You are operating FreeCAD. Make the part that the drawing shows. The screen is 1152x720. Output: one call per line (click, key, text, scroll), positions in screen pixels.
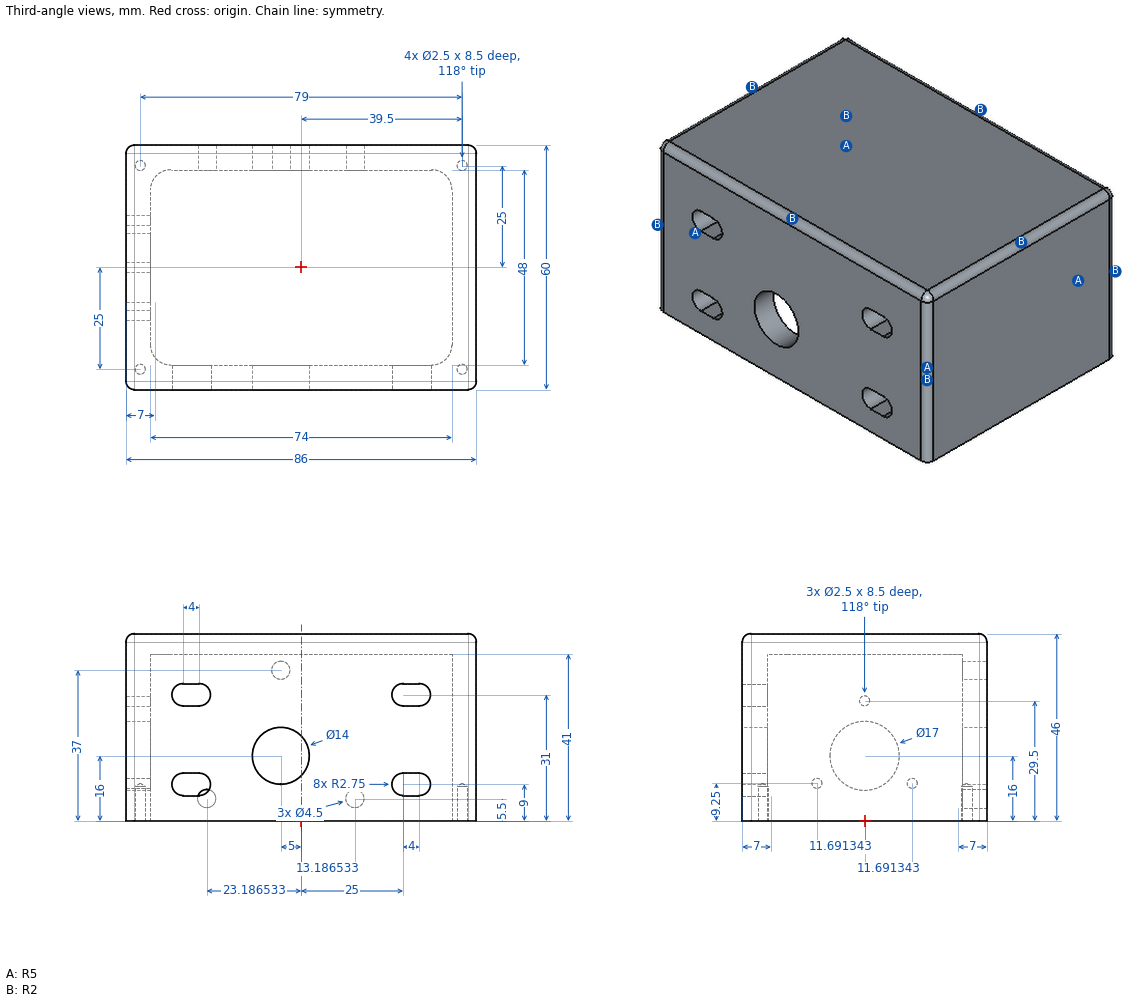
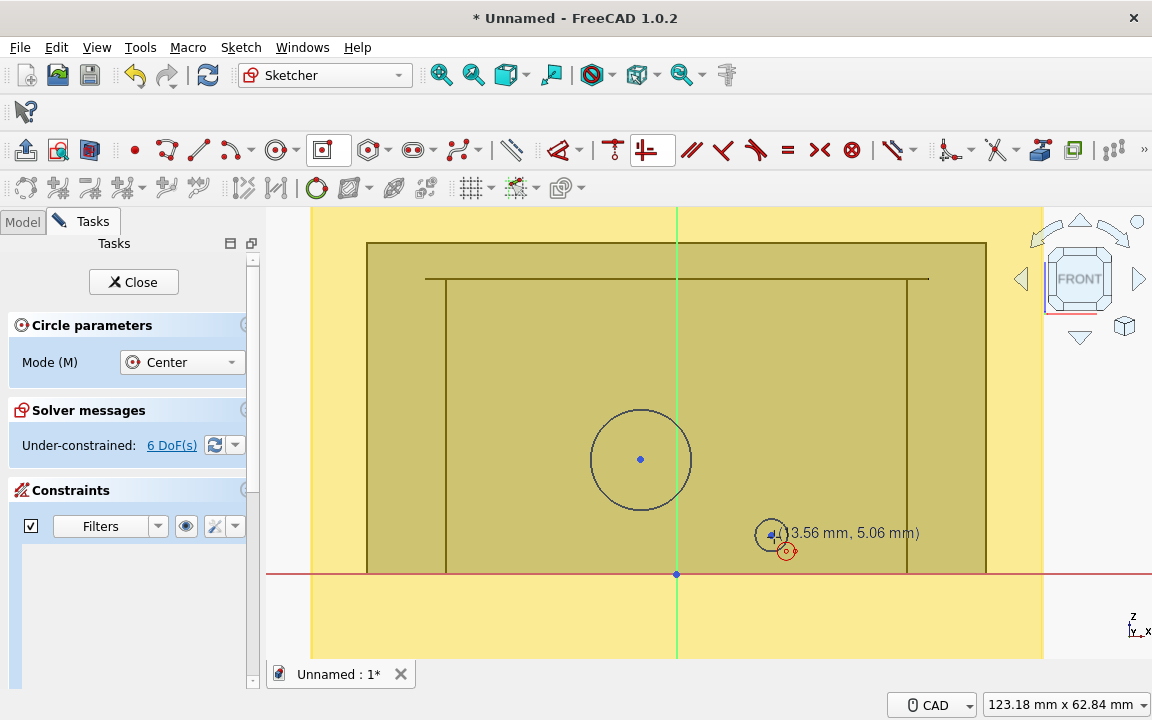
scroll(641, 308, up, 2)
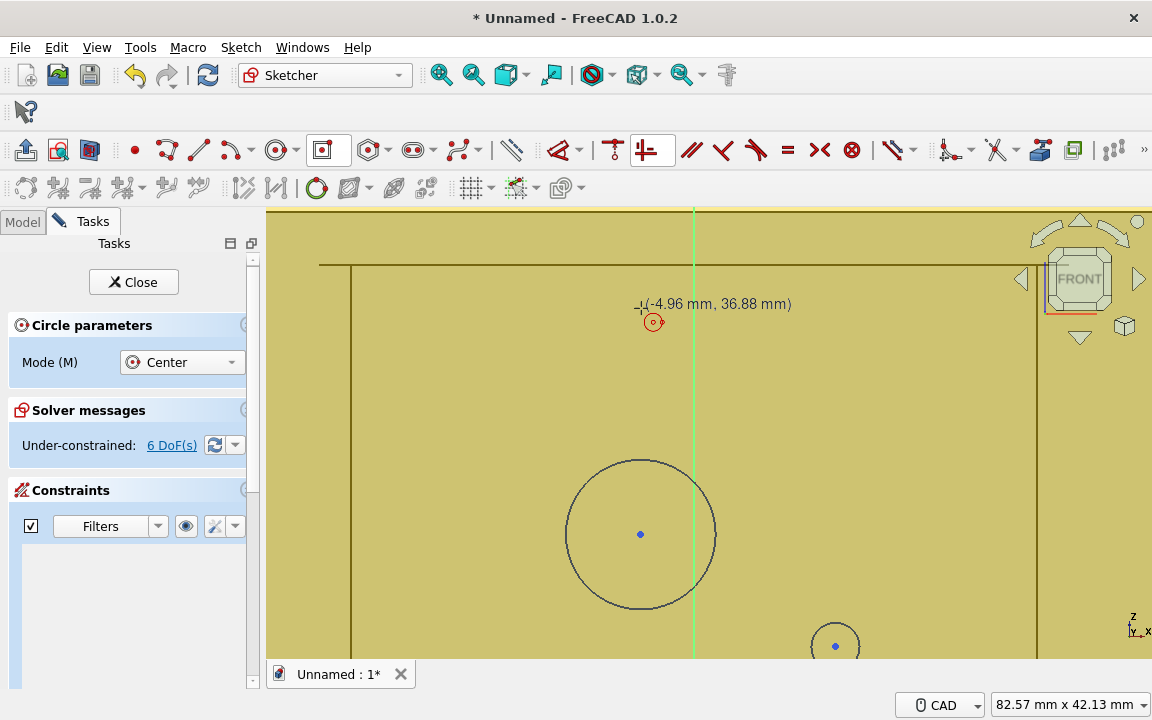
click(640, 308)
click(657, 291)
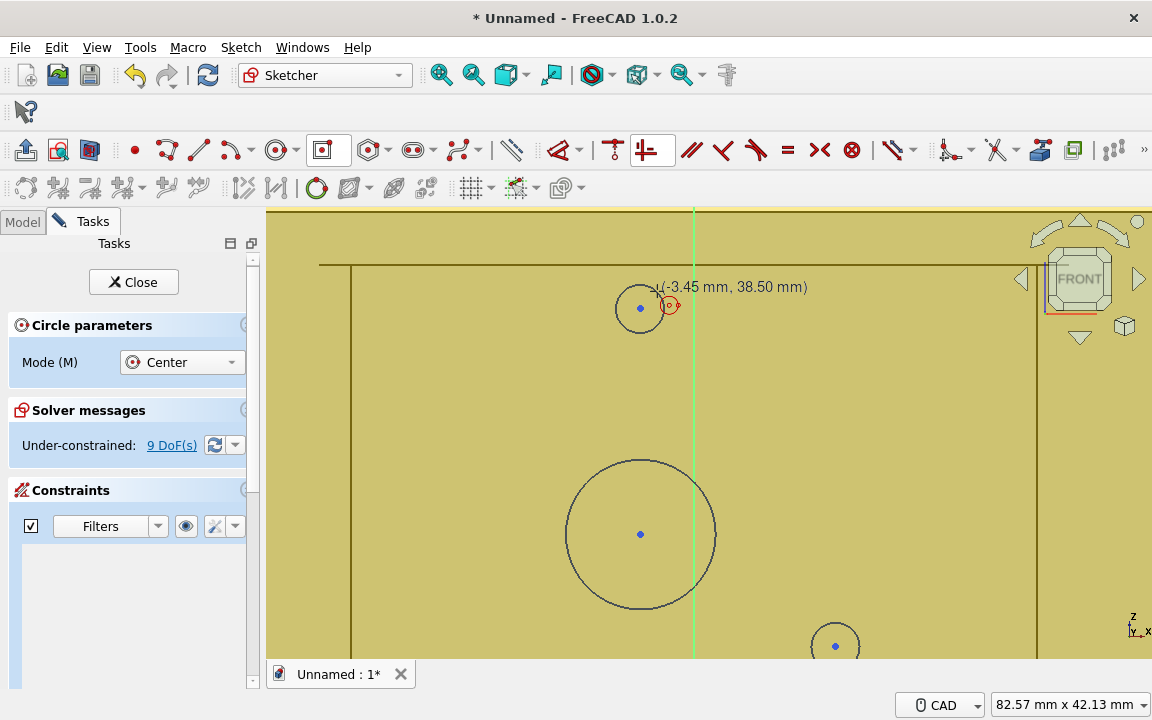
scroll(641, 308, down, 2)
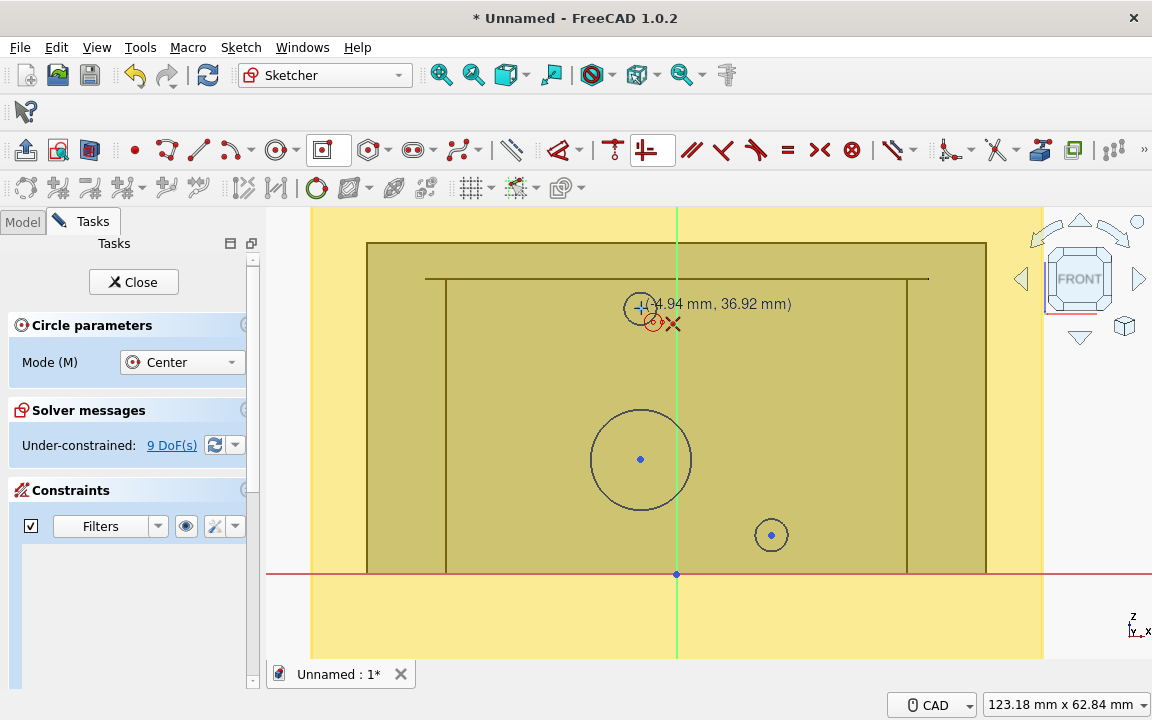
scroll(510, 535, up, 2)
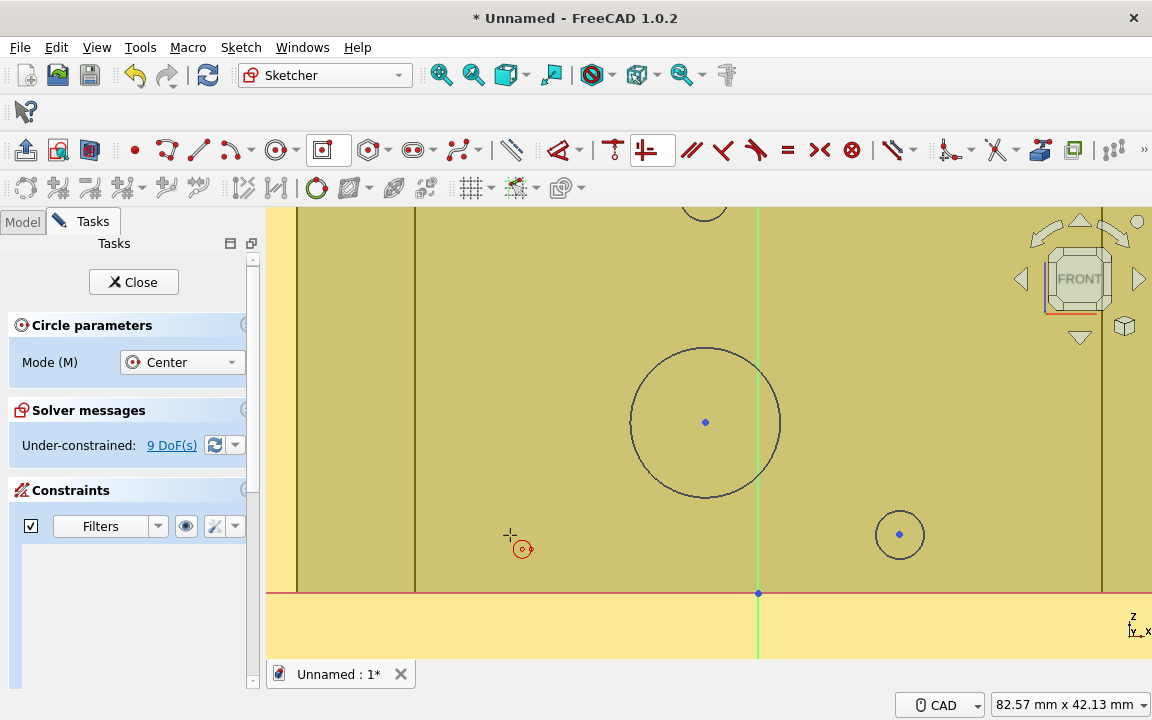
click(510, 534)
click(527, 517)
key(Escape)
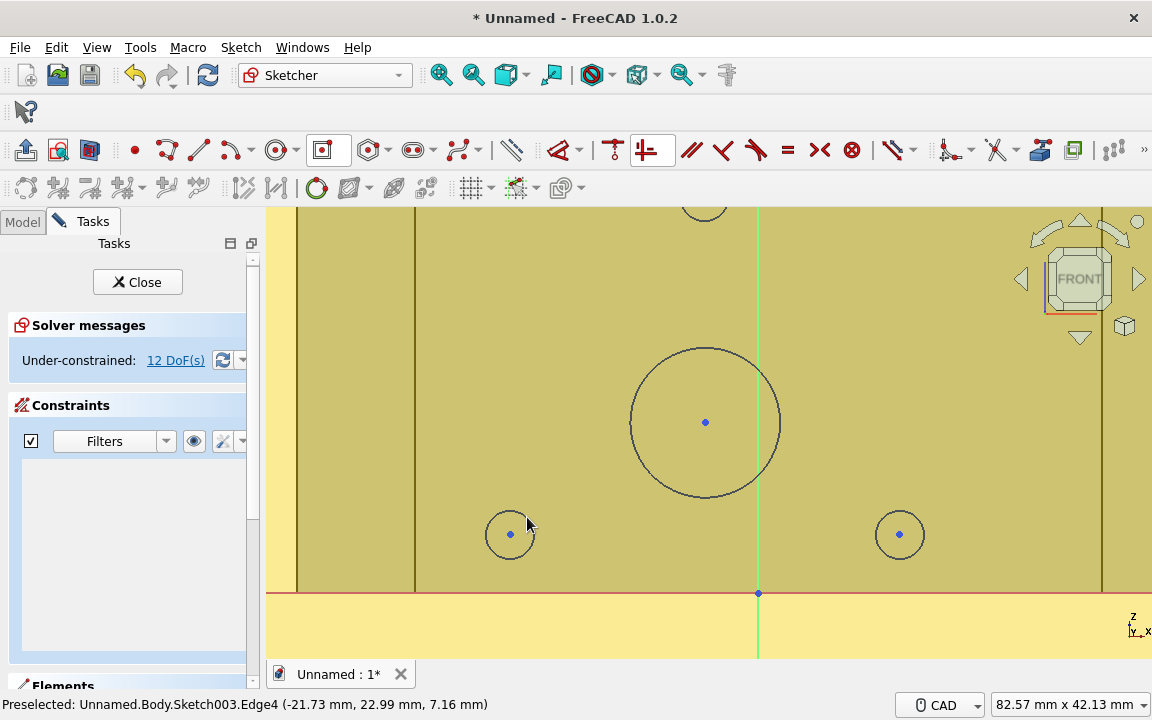
click(917, 518)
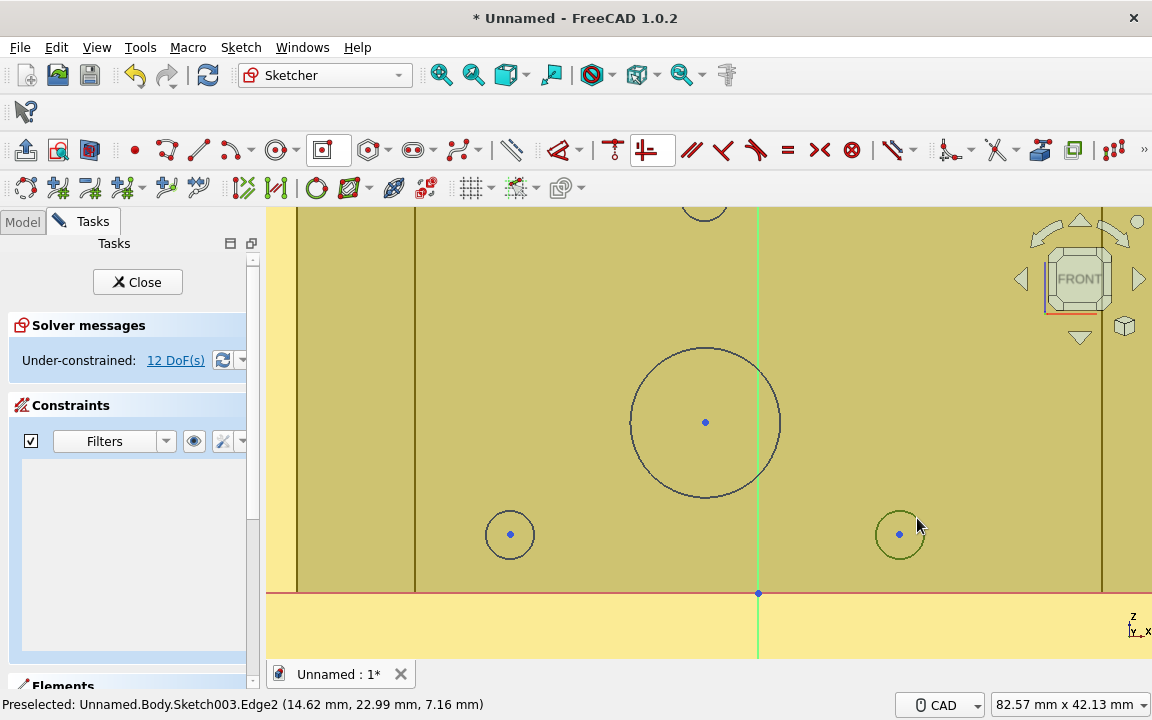
scroll(510, 535, down, 2)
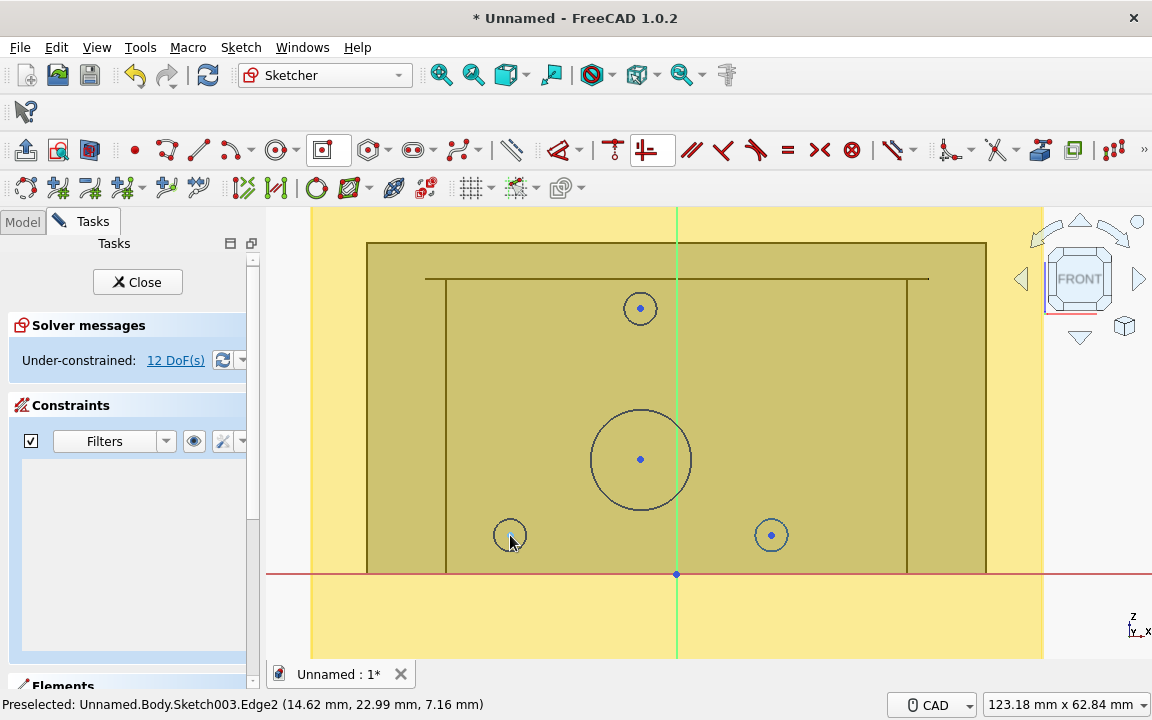
click(652, 297)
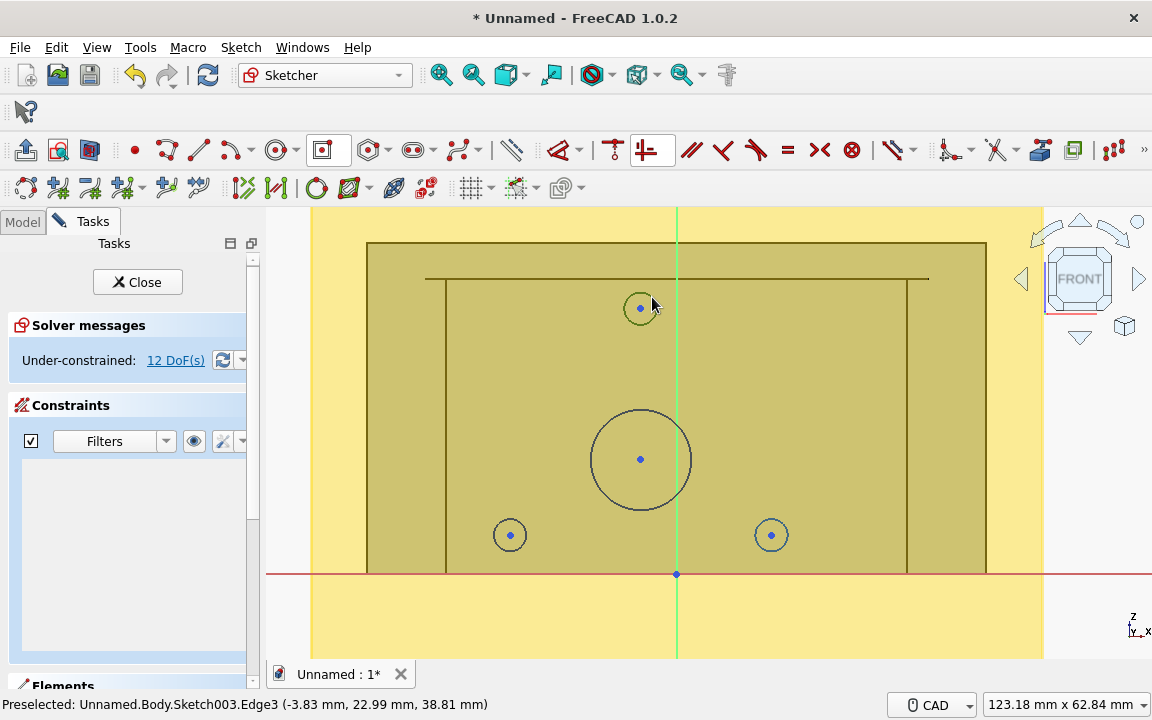
click(521, 524)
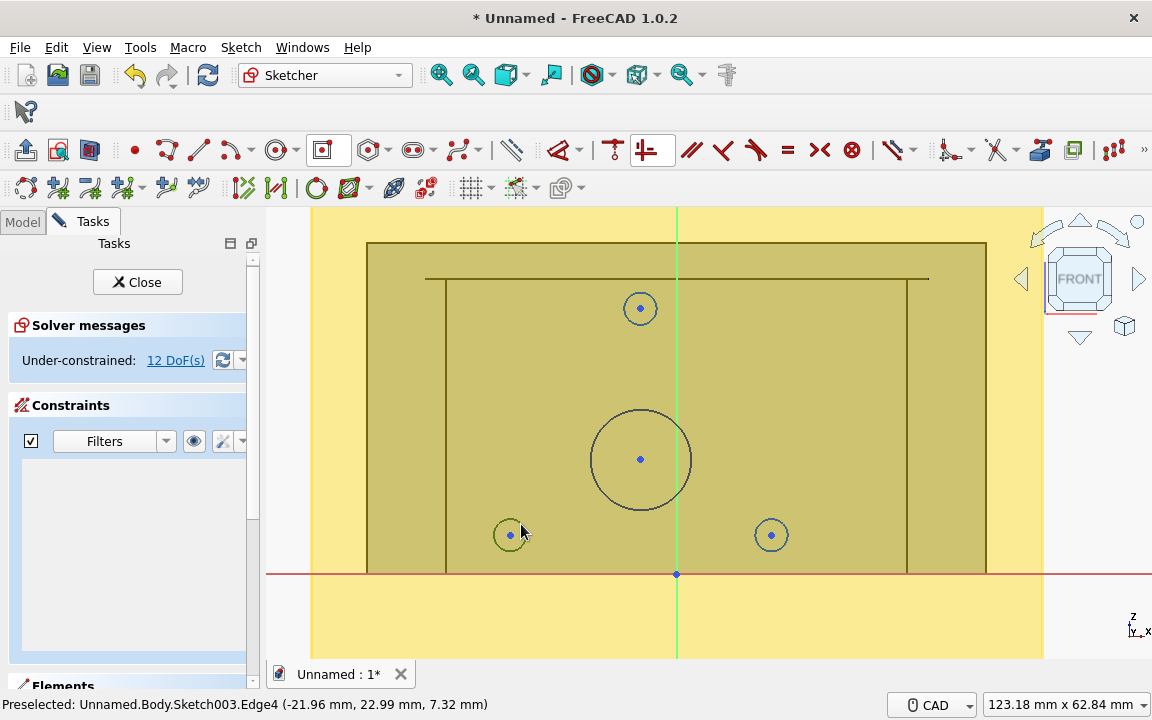
key(e)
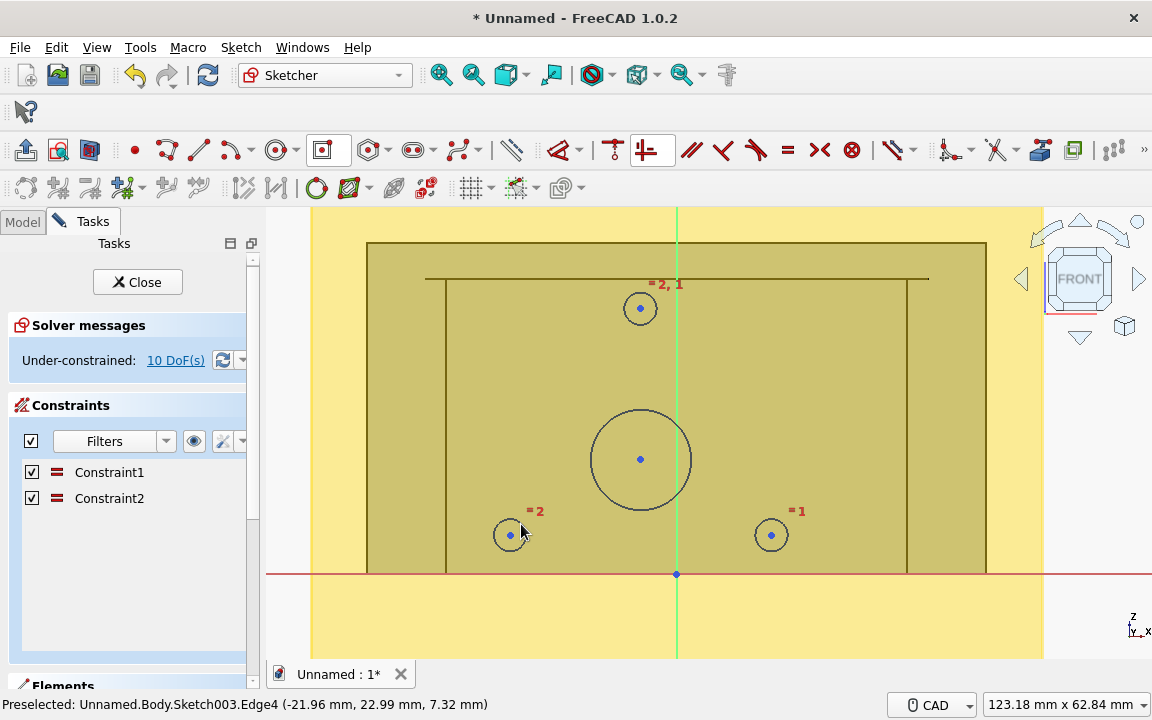
click(641, 460)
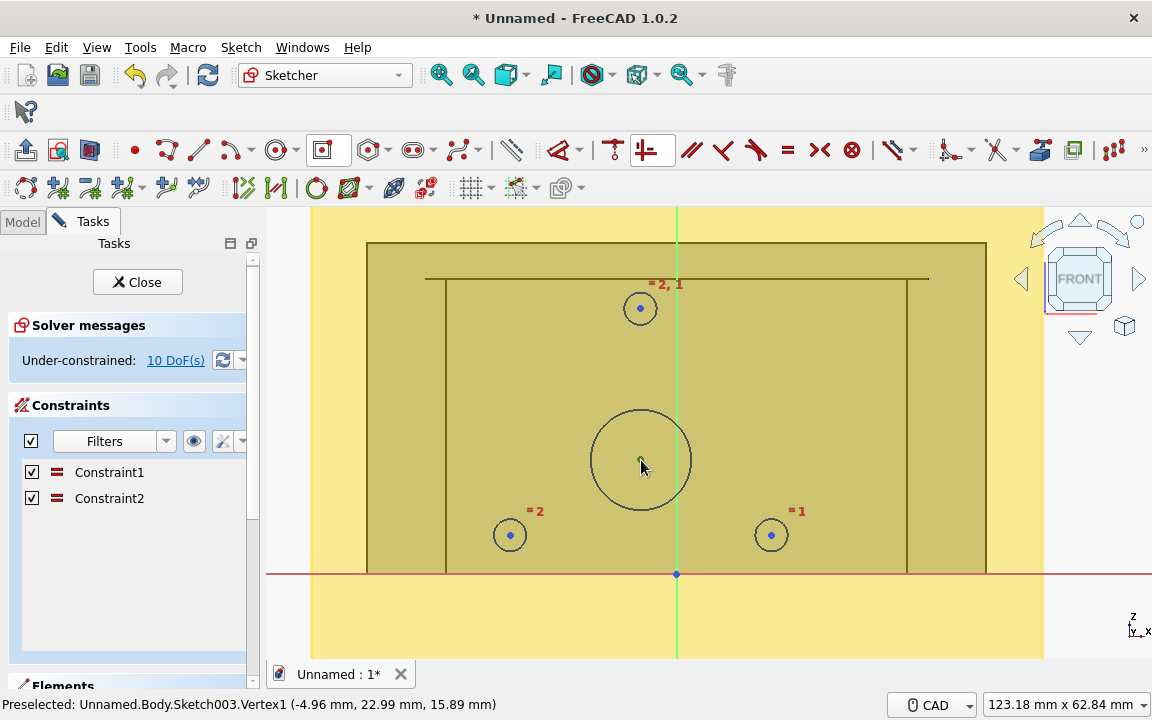
click(640, 309)